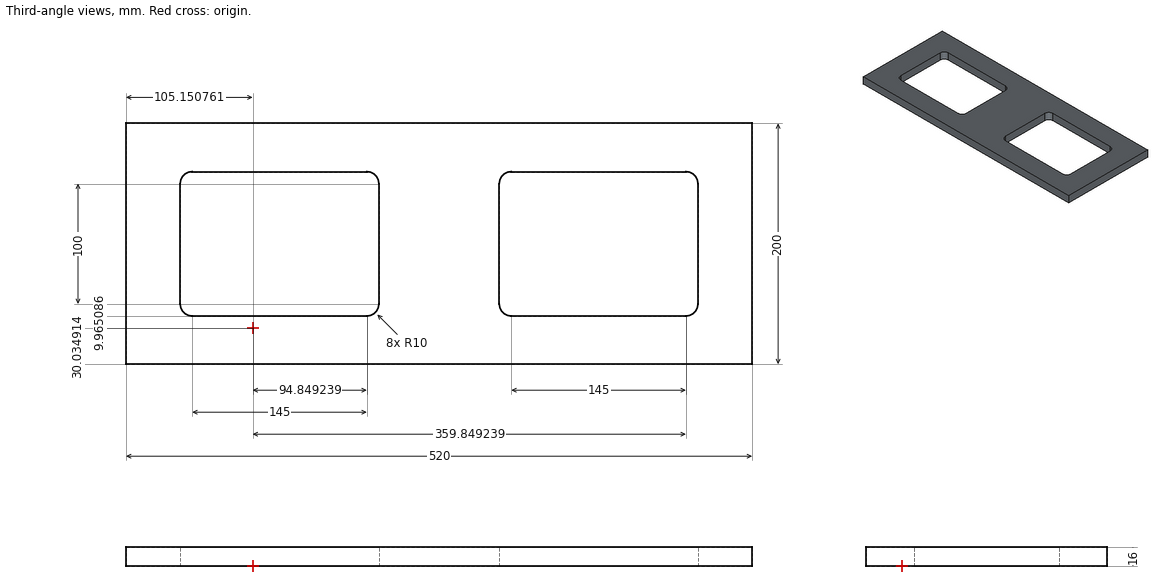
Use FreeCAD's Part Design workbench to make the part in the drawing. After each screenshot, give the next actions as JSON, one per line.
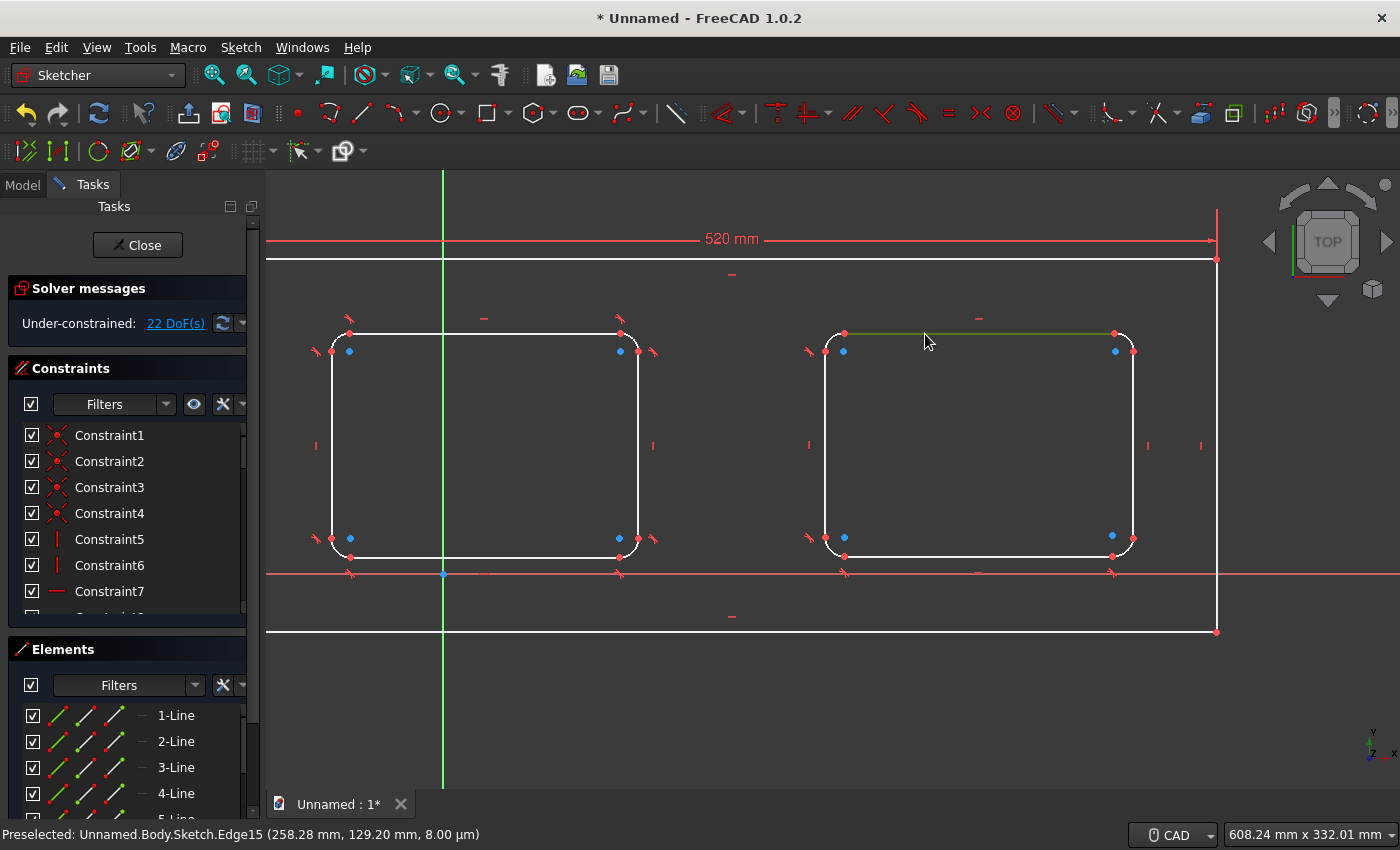
{"action": "left_click", "coordinate": [831, 338]}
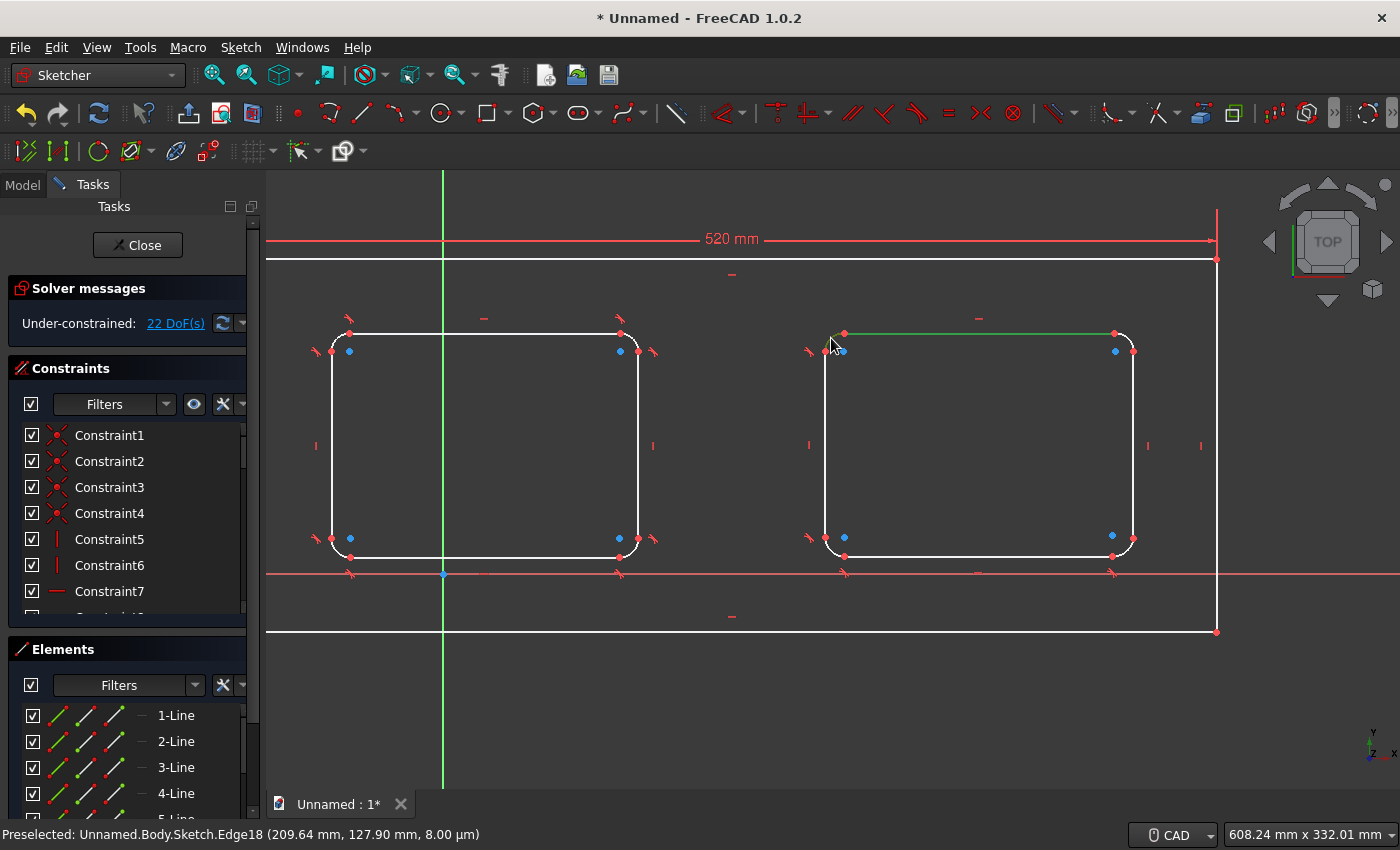
{"action": "key", "text": "t"}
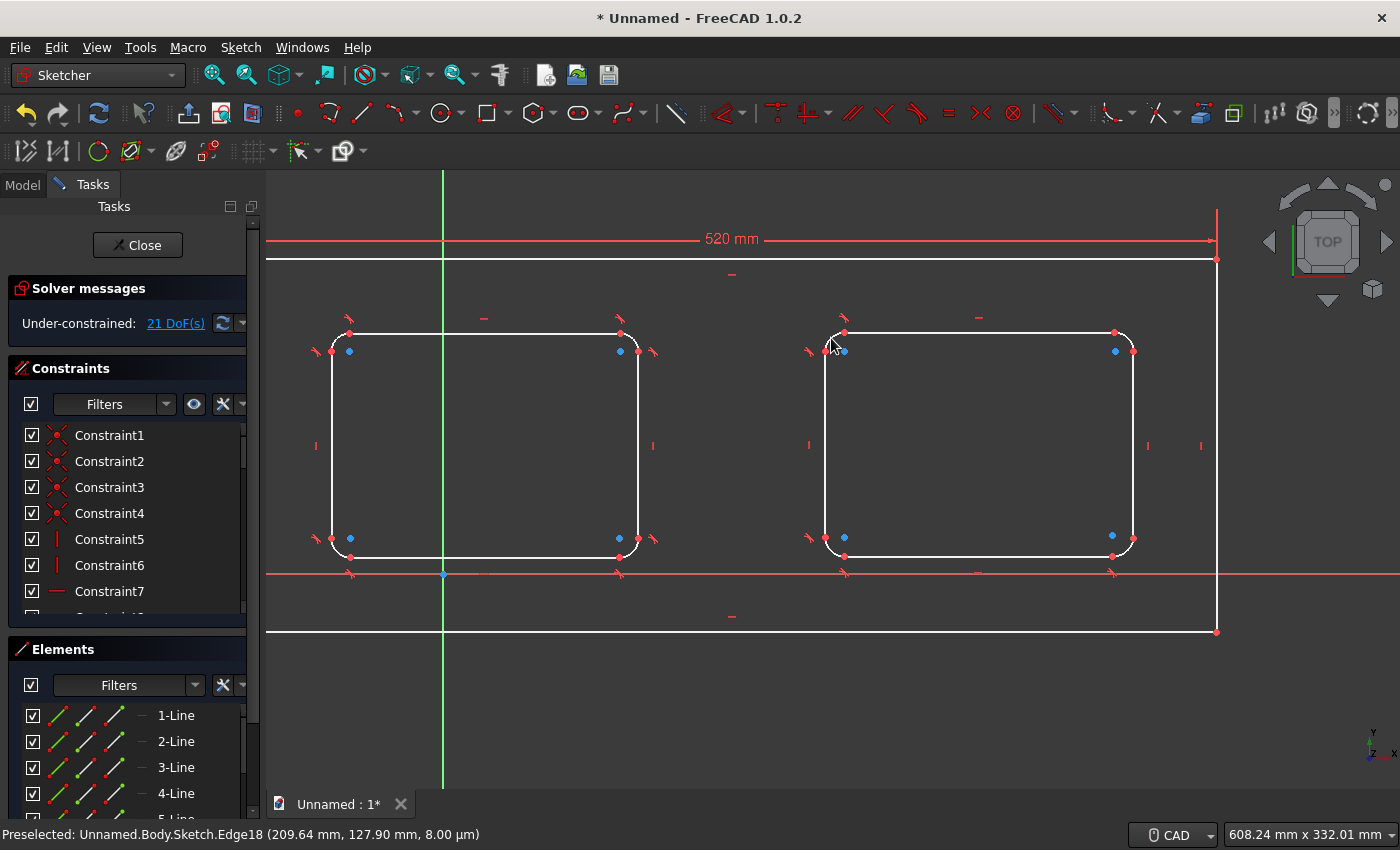
{"action": "left_click", "coordinate": [925, 333]}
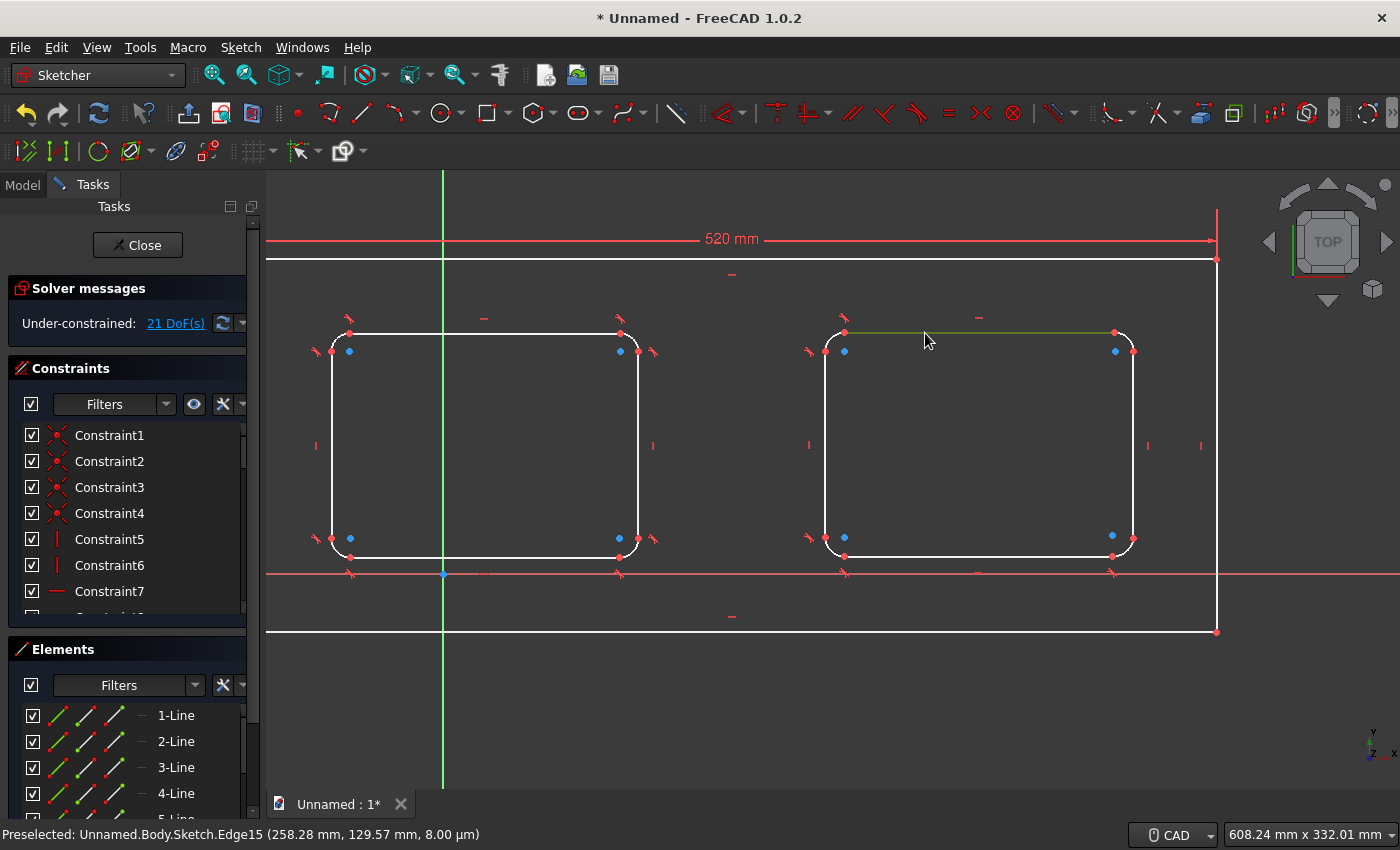
{"action": "left_click", "coordinate": [1128, 338]}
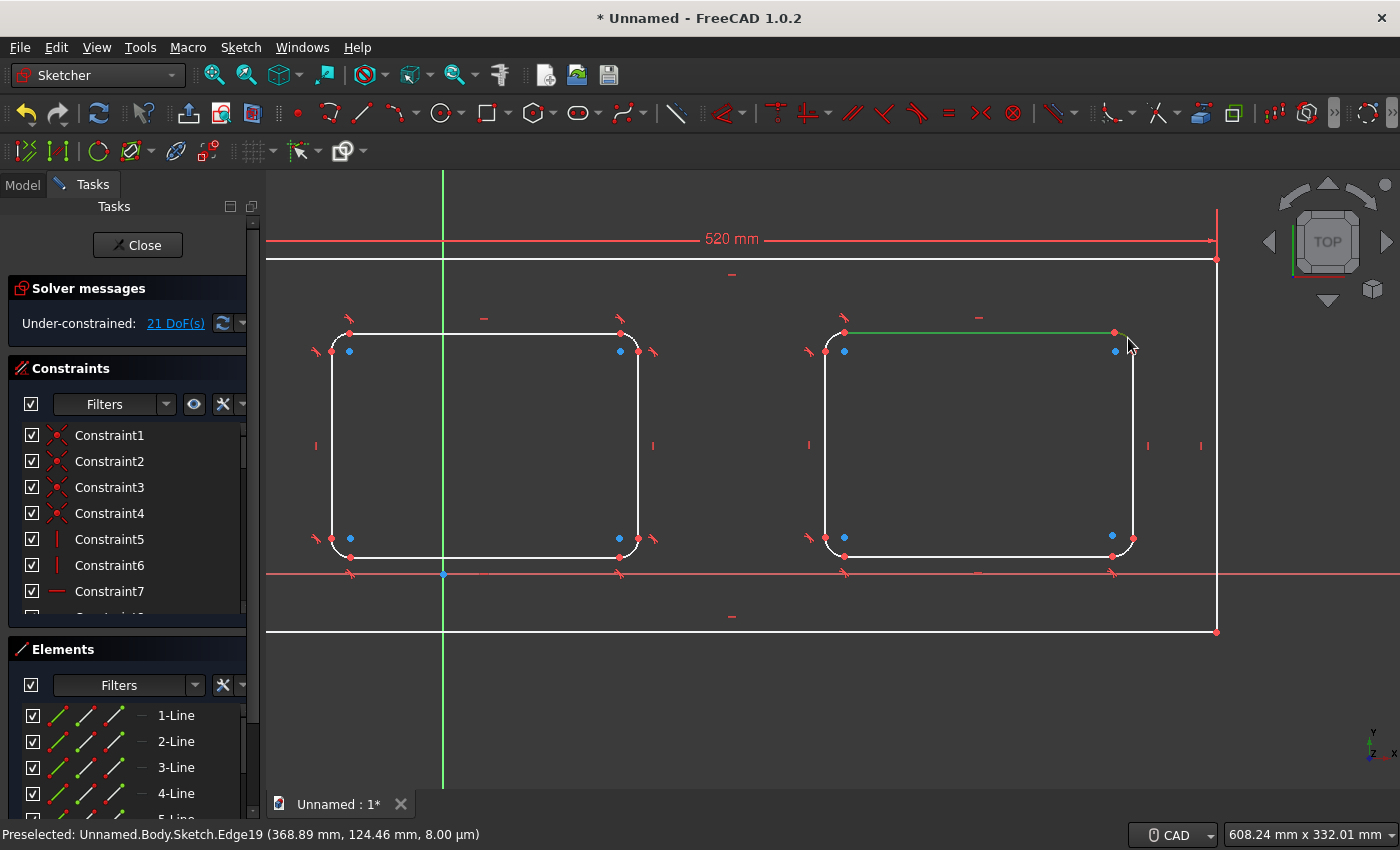
{"action": "key", "text": "t"}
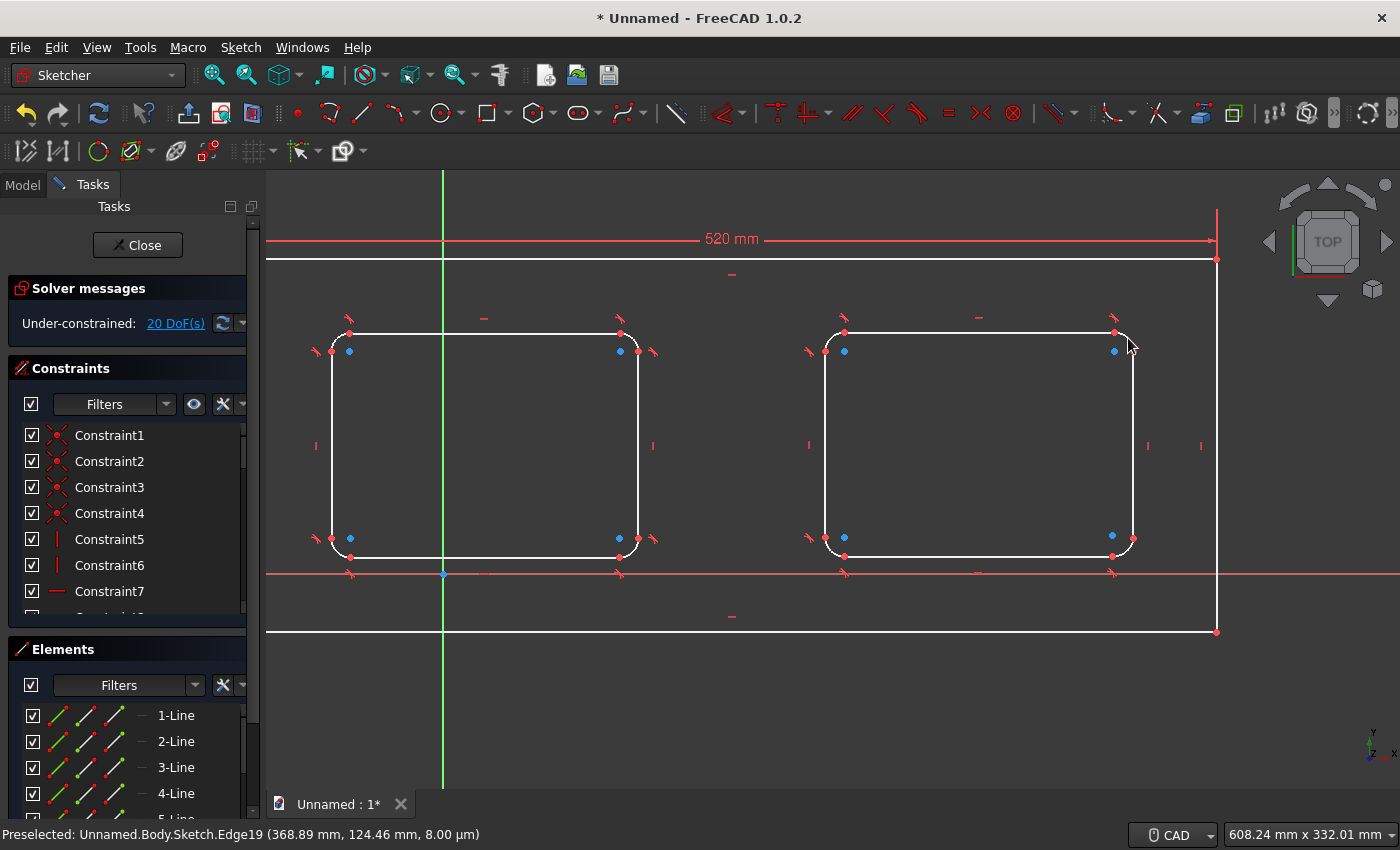
{"action": "left_click", "coordinate": [1133, 408]}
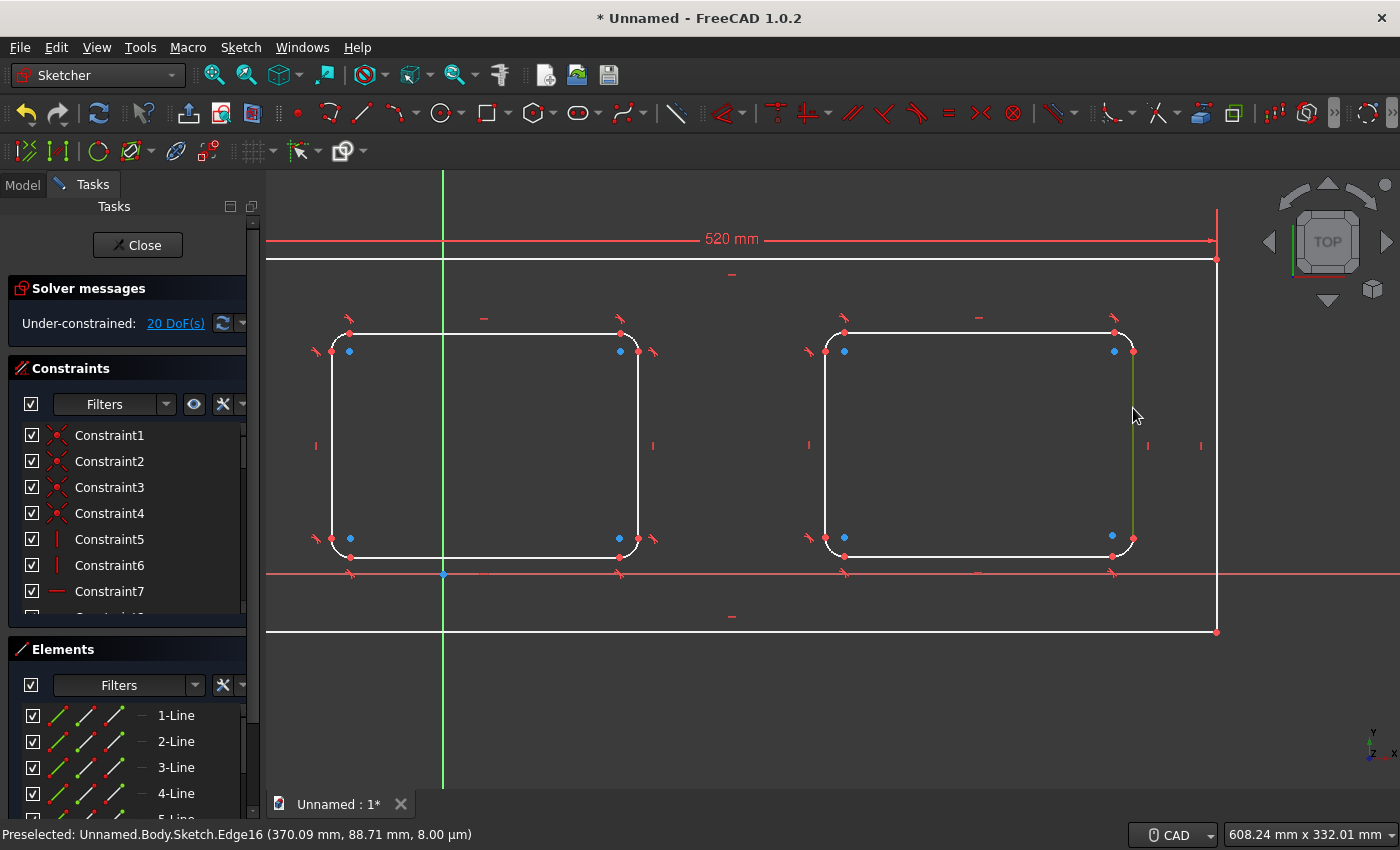
{"action": "left_click", "coordinate": [1128, 338]}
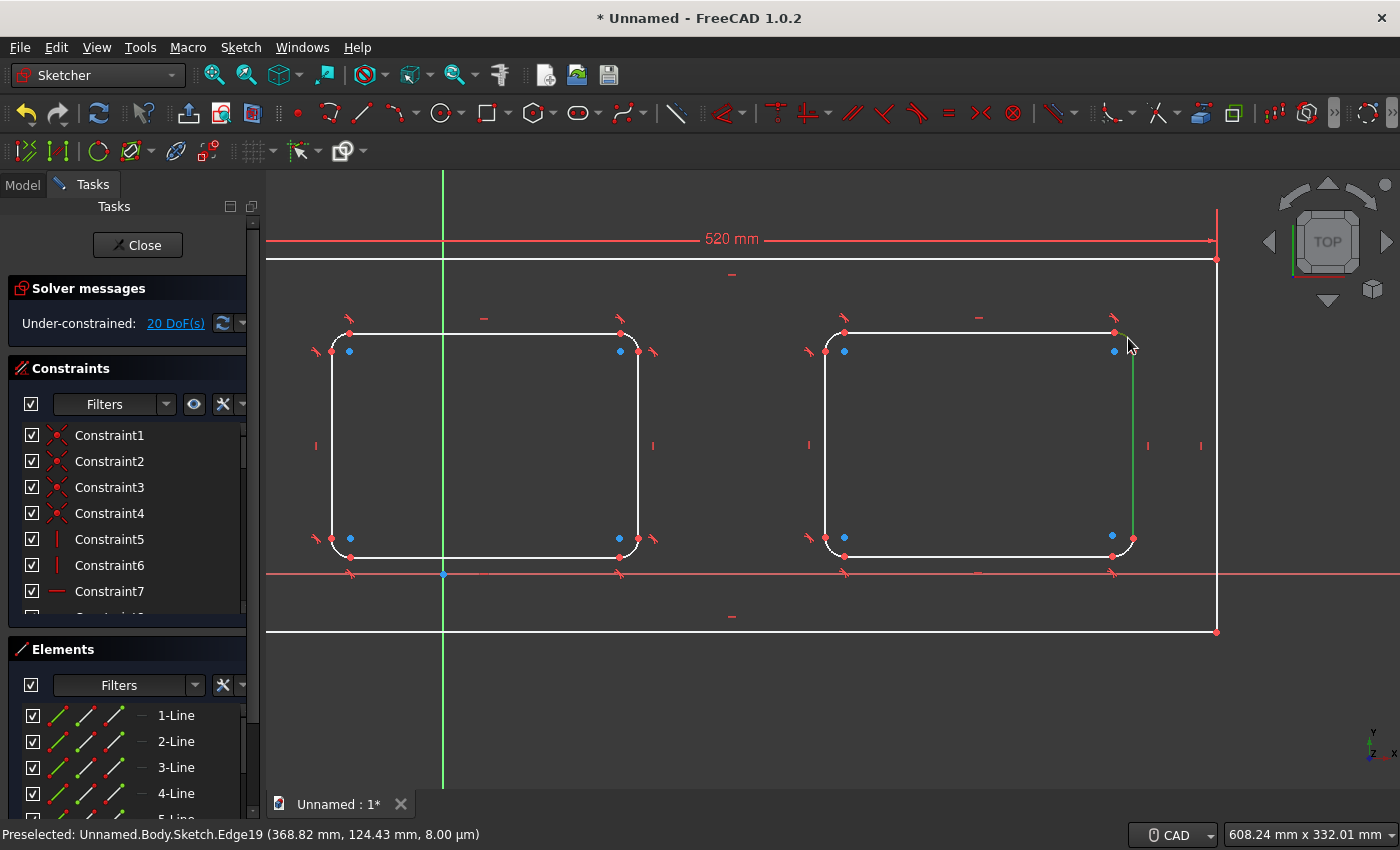
{"action": "left_click", "coordinate": [918, 114]}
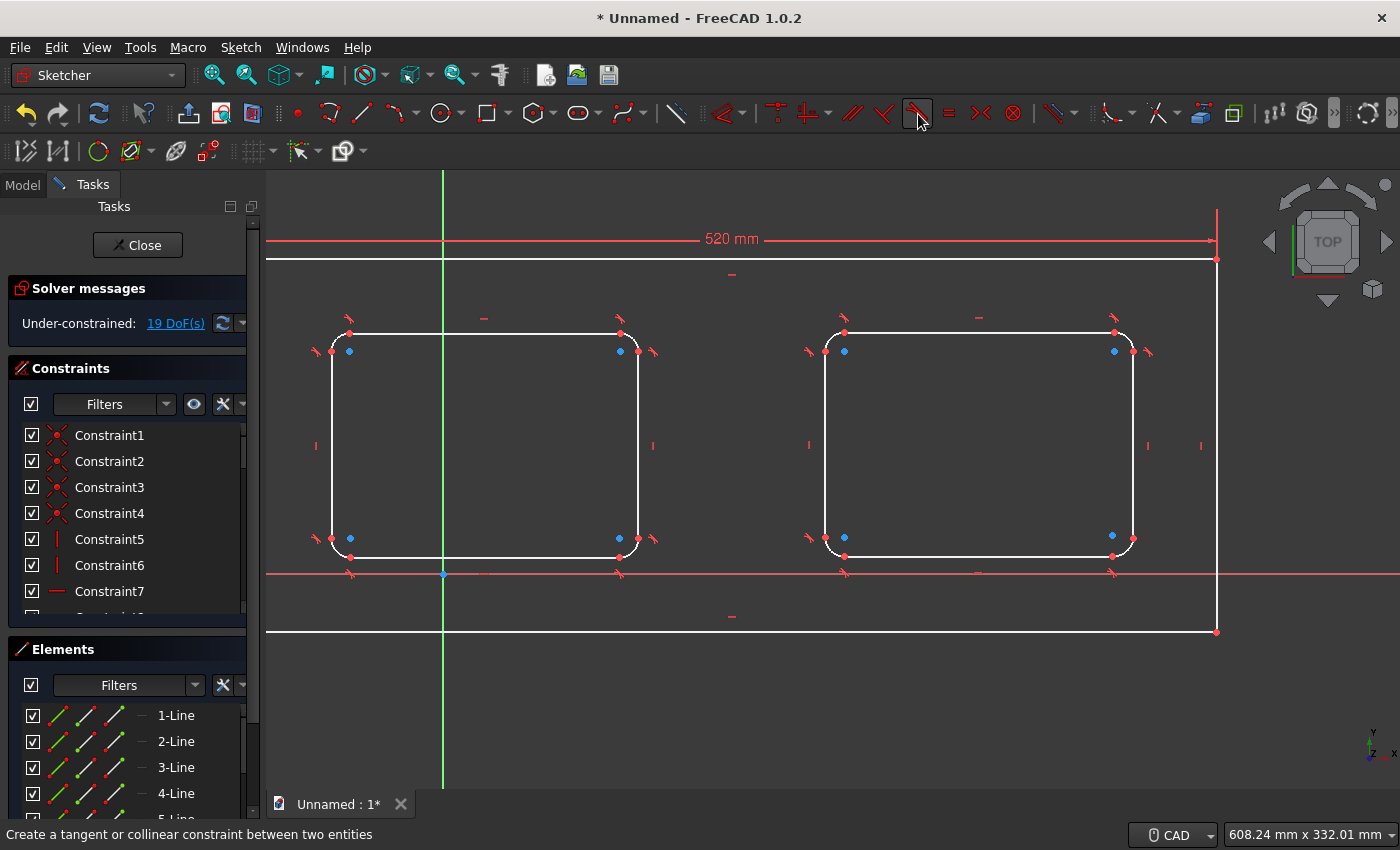
{"action": "left_click", "coordinate": [1133, 408]}